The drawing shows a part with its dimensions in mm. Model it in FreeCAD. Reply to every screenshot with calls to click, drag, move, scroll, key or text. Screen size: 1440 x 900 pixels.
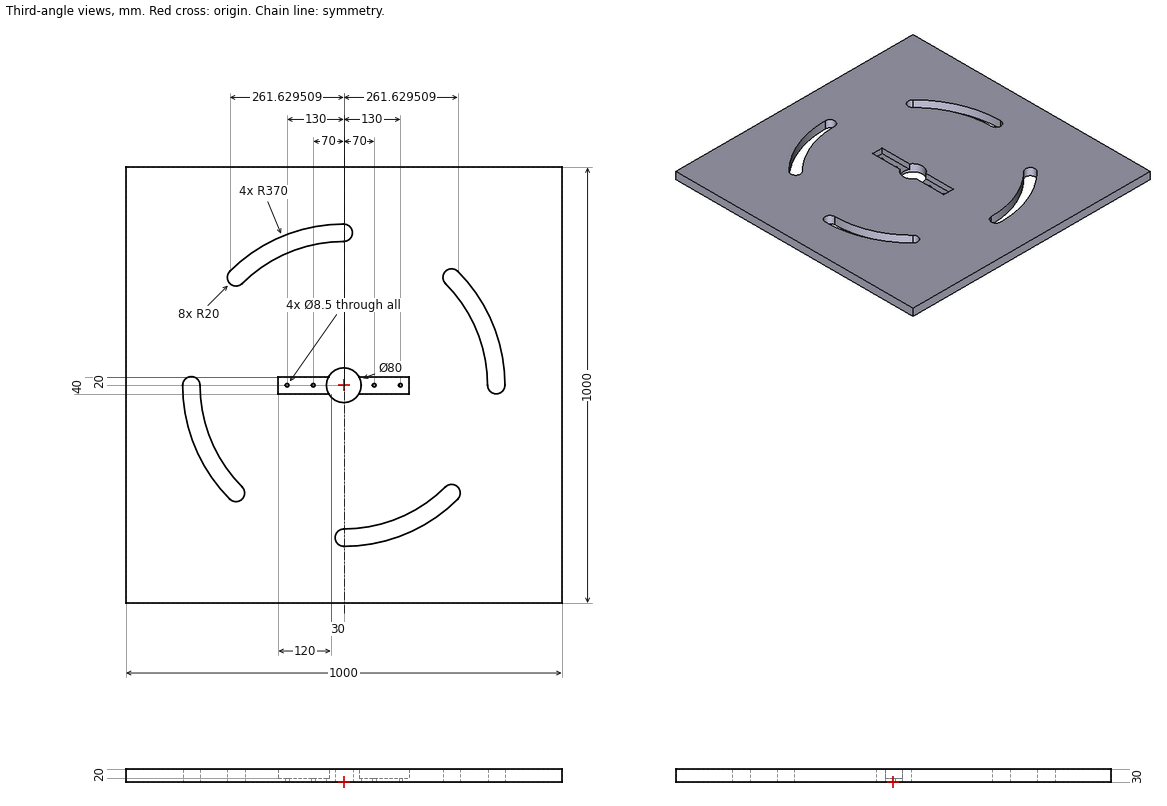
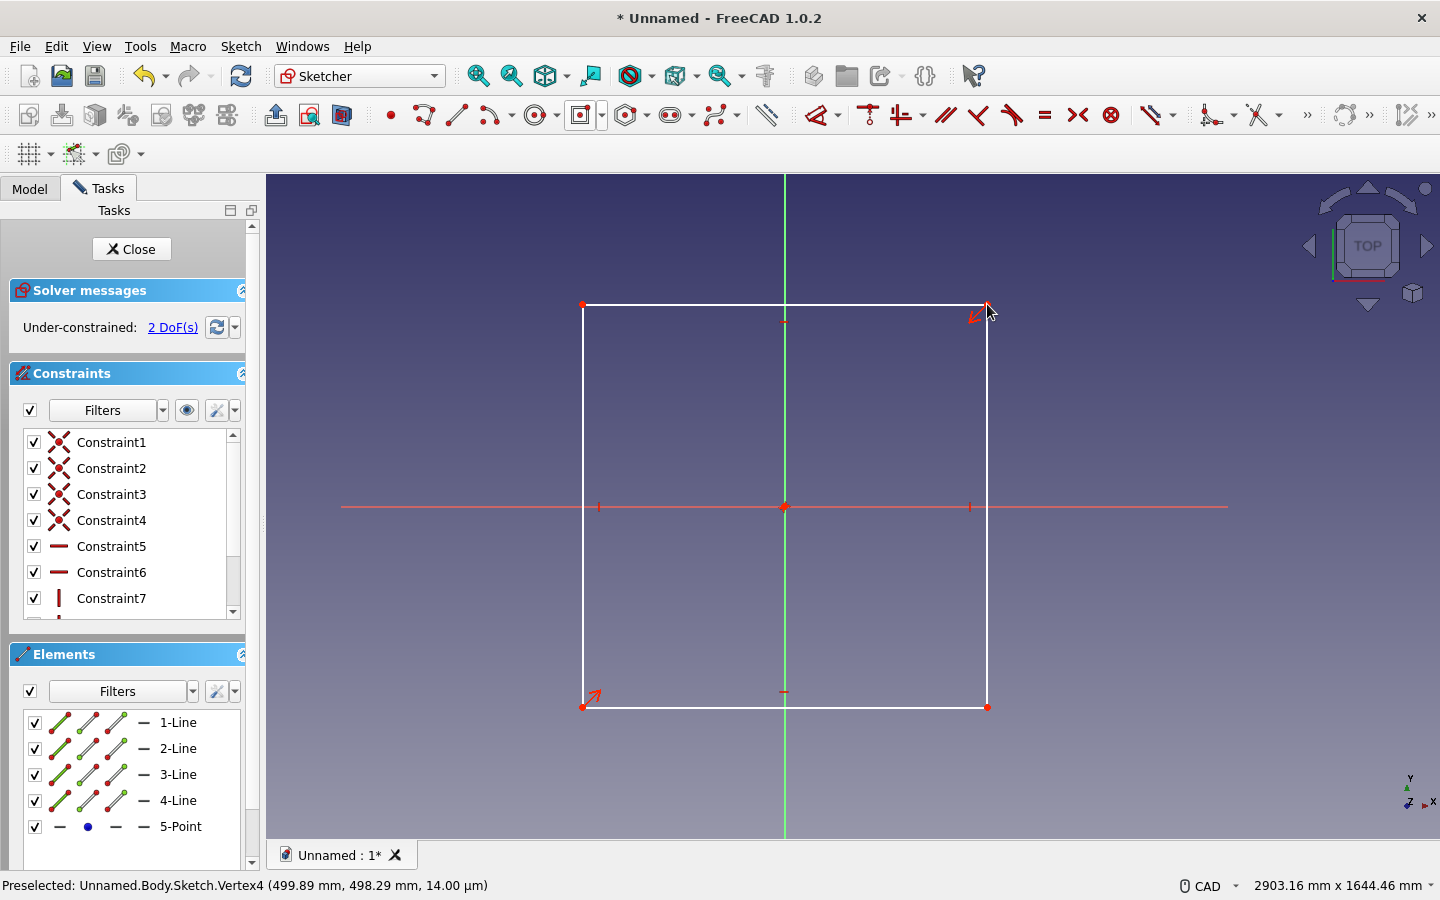
click(816, 116)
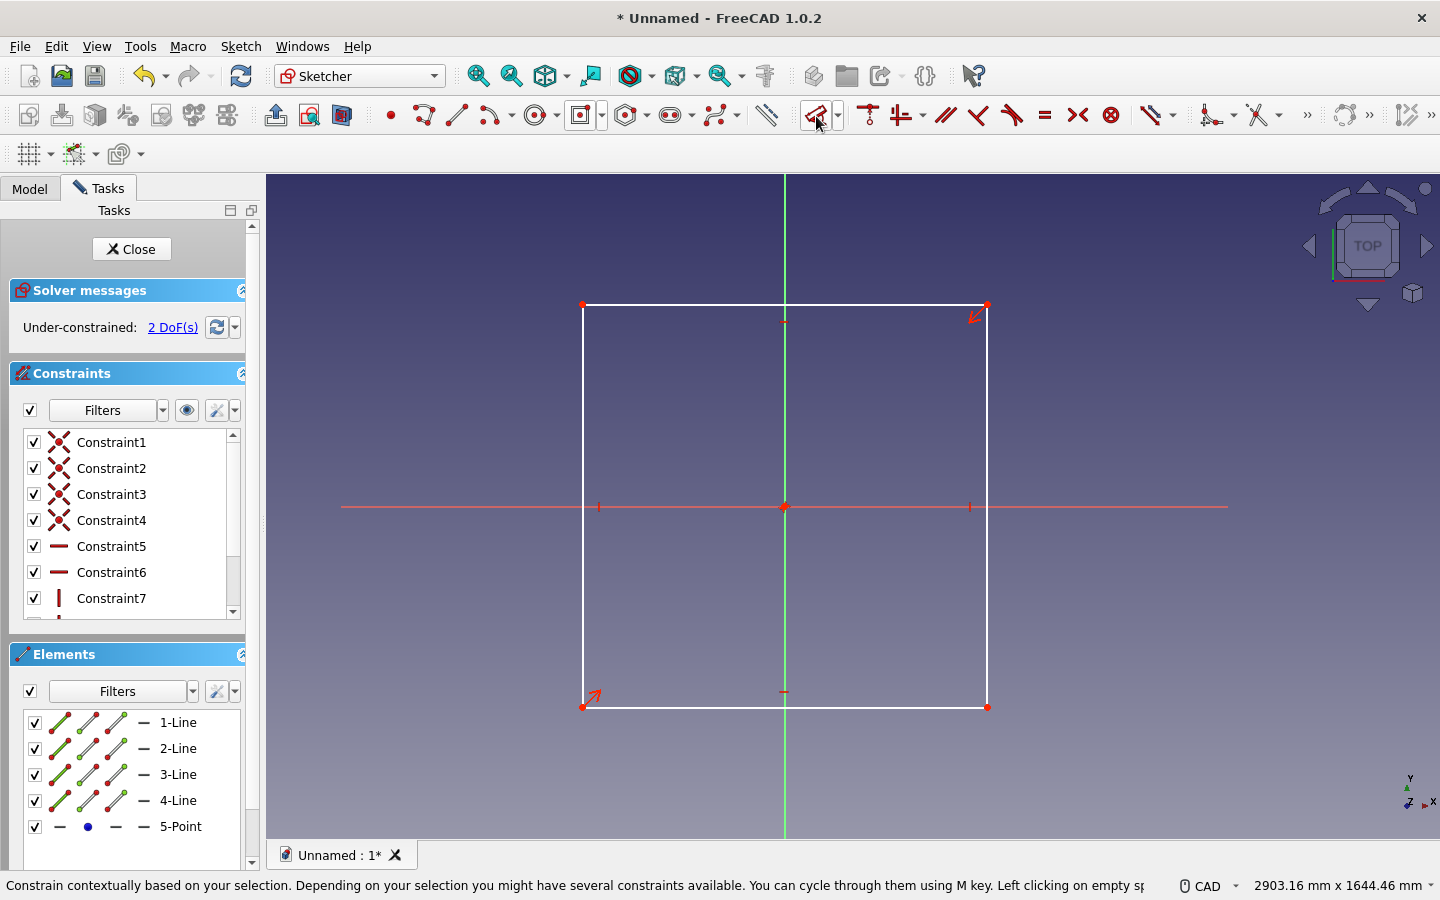
click(704, 708)
click(692, 742)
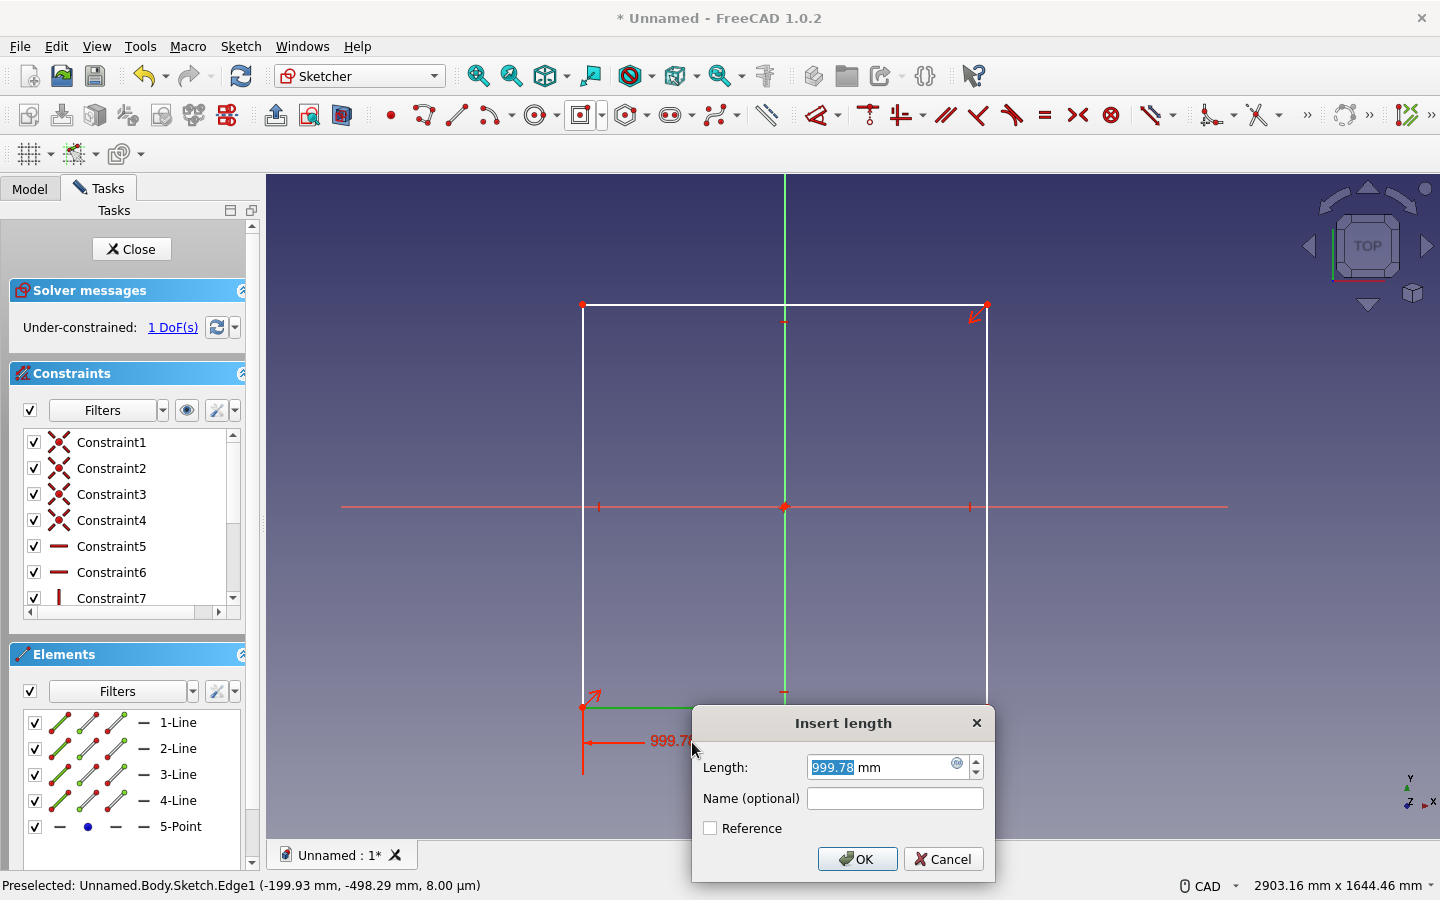
text(1000)
key(Return)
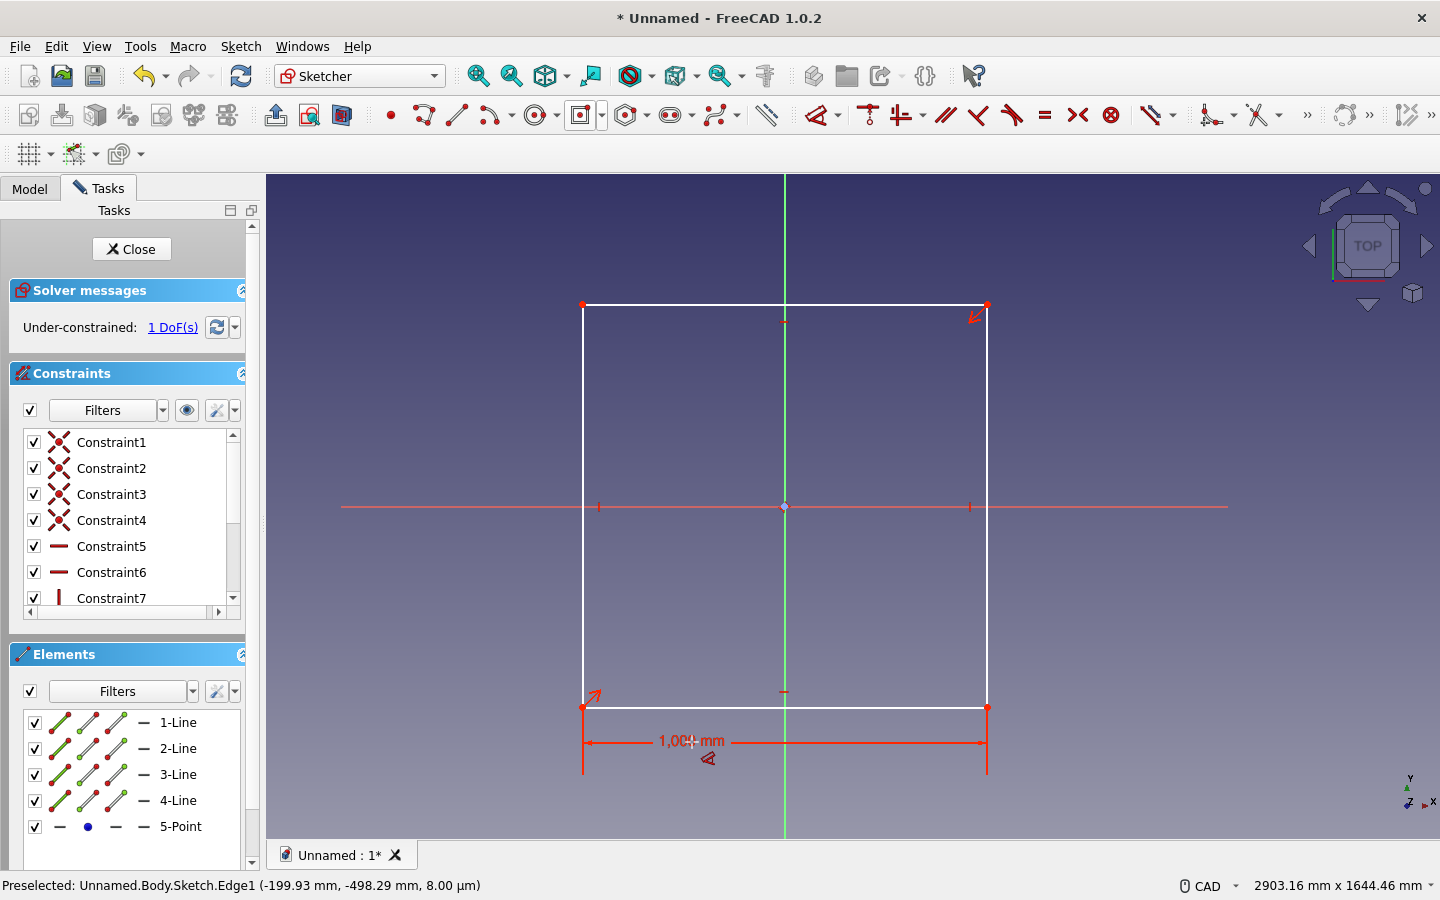
click(987, 587)
click(1021, 414)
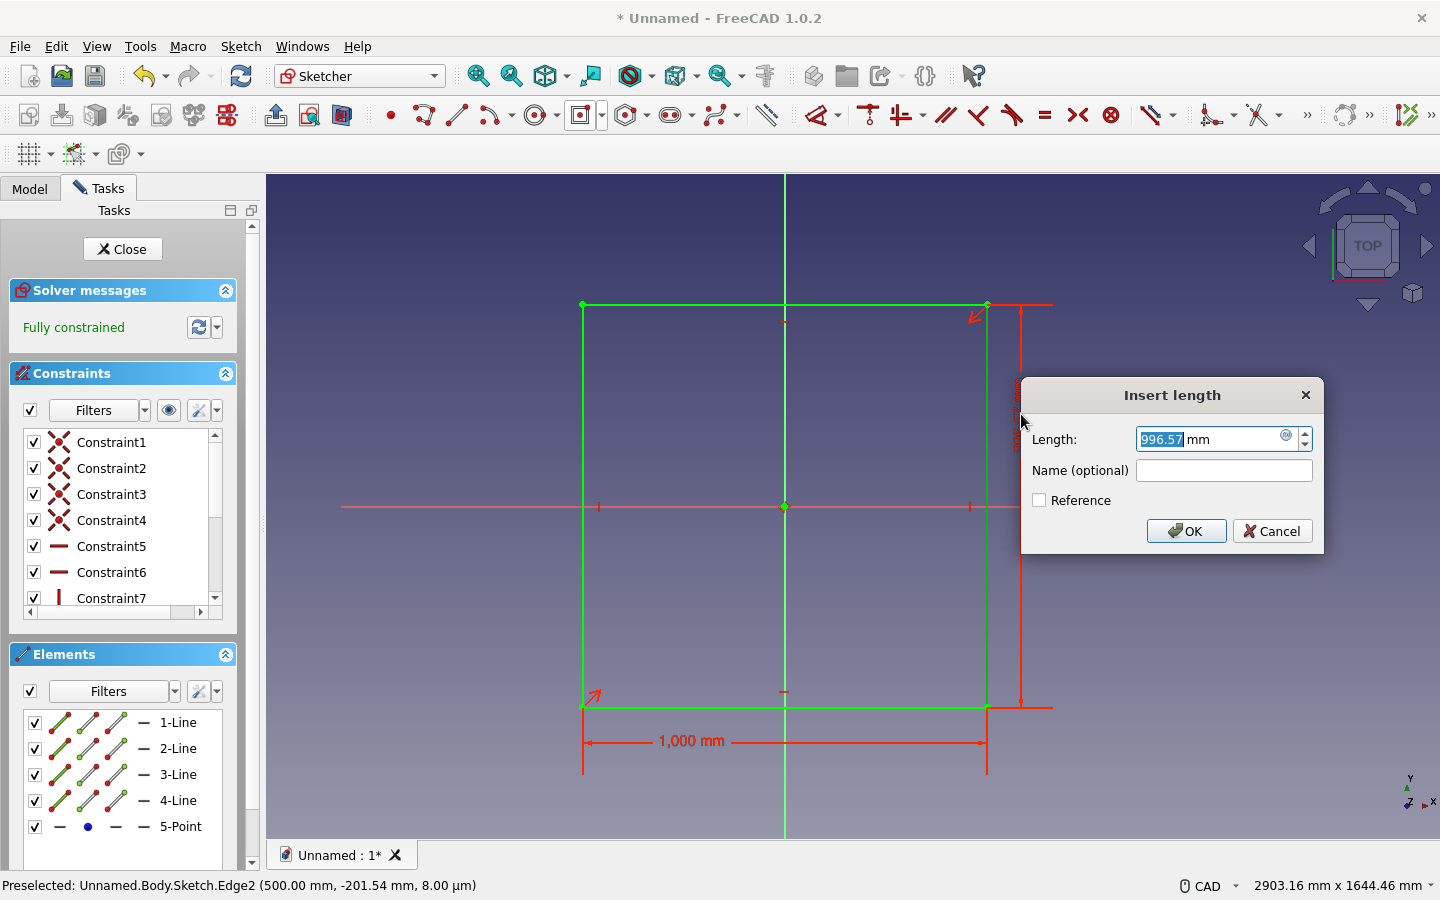
text(1000)
key(Return)
key(Escape)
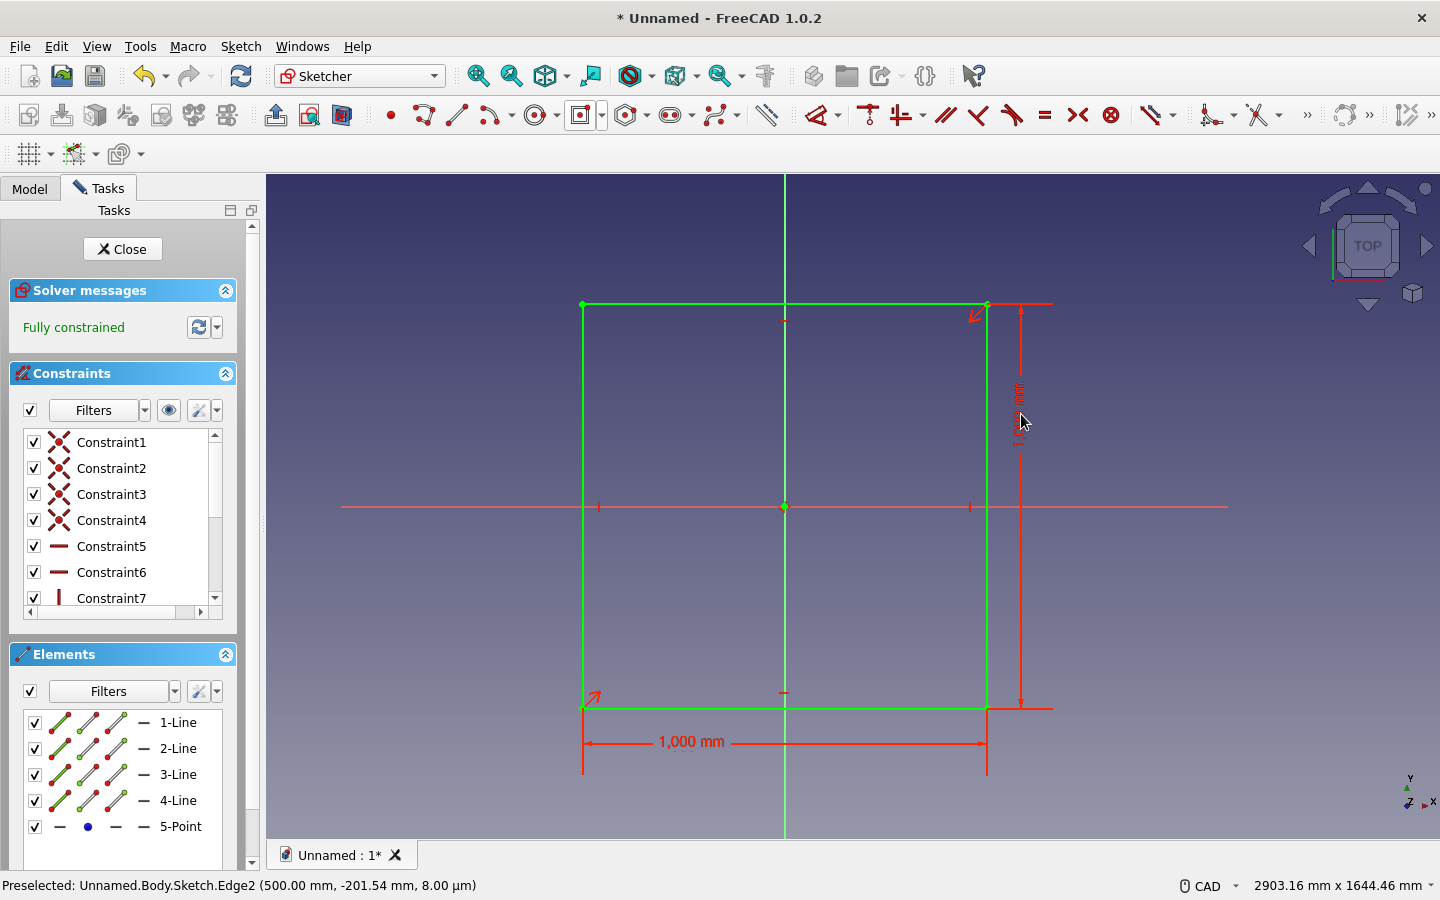
click(123, 249)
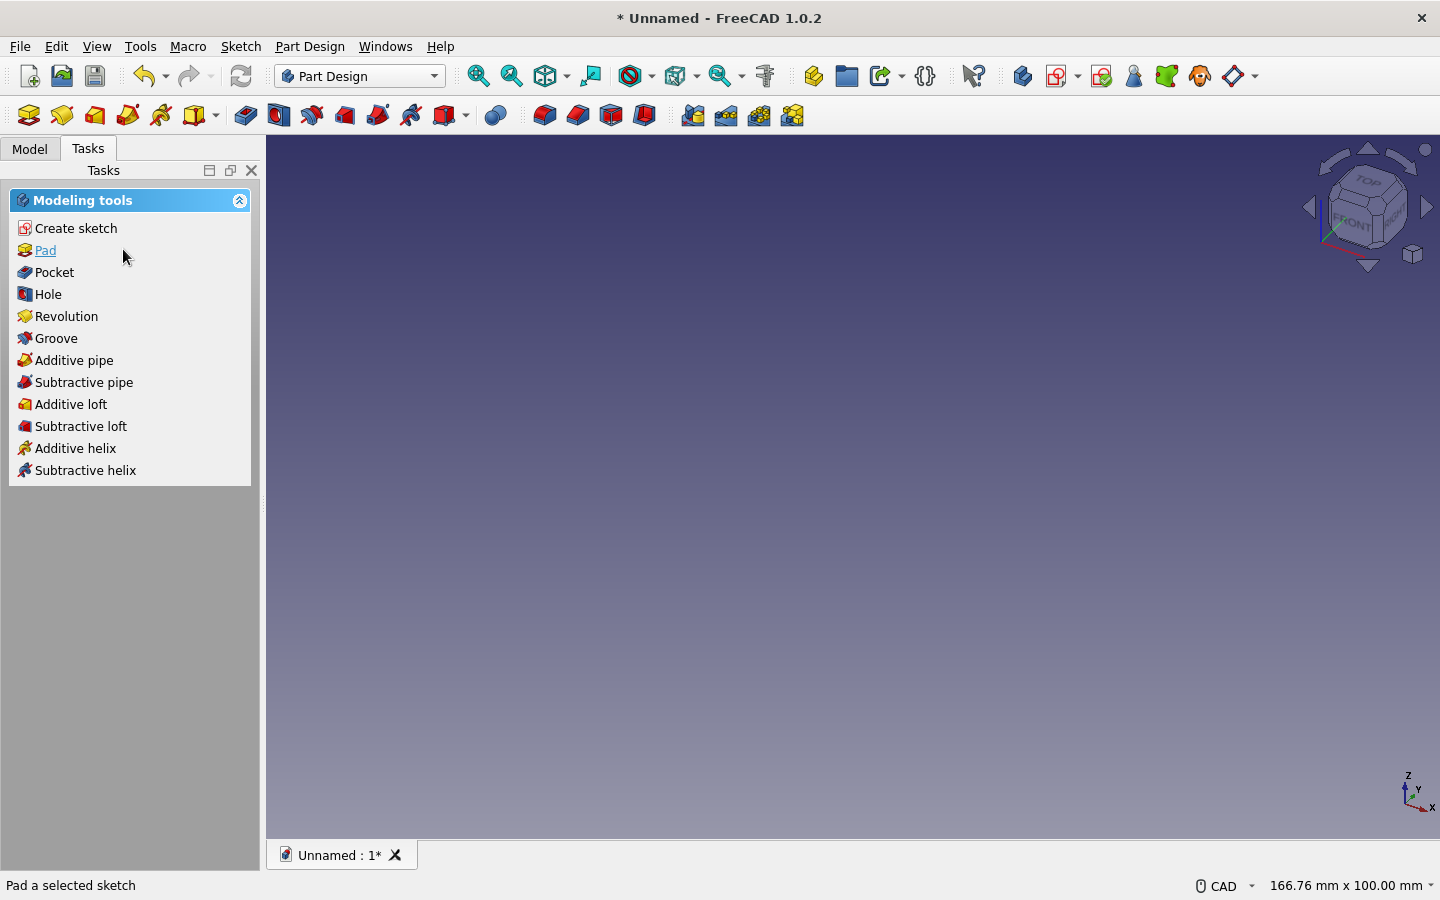
click(29, 116)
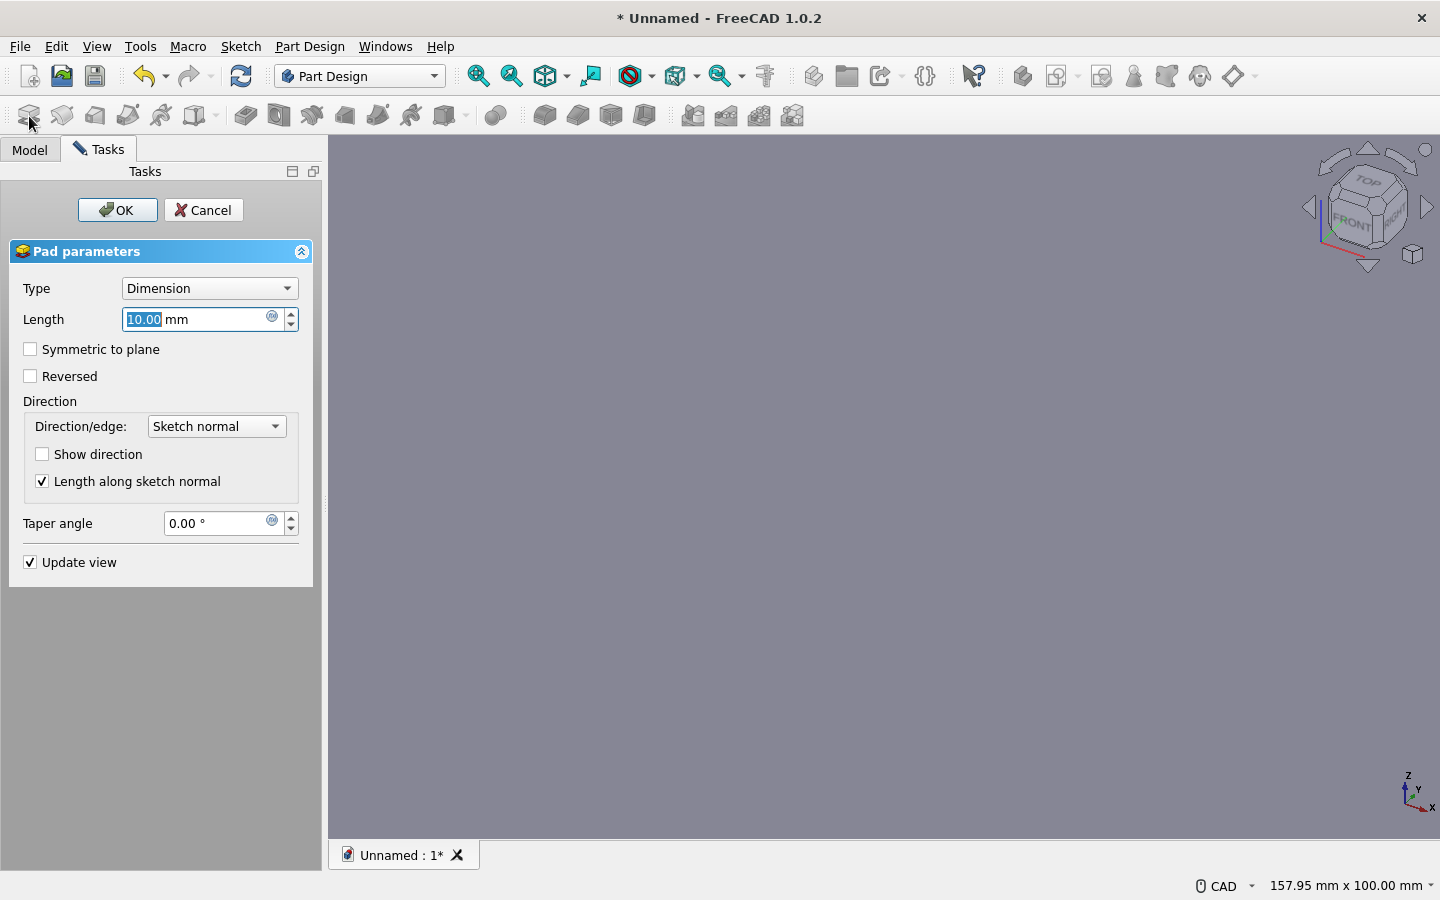
text(30)
key(Tab)